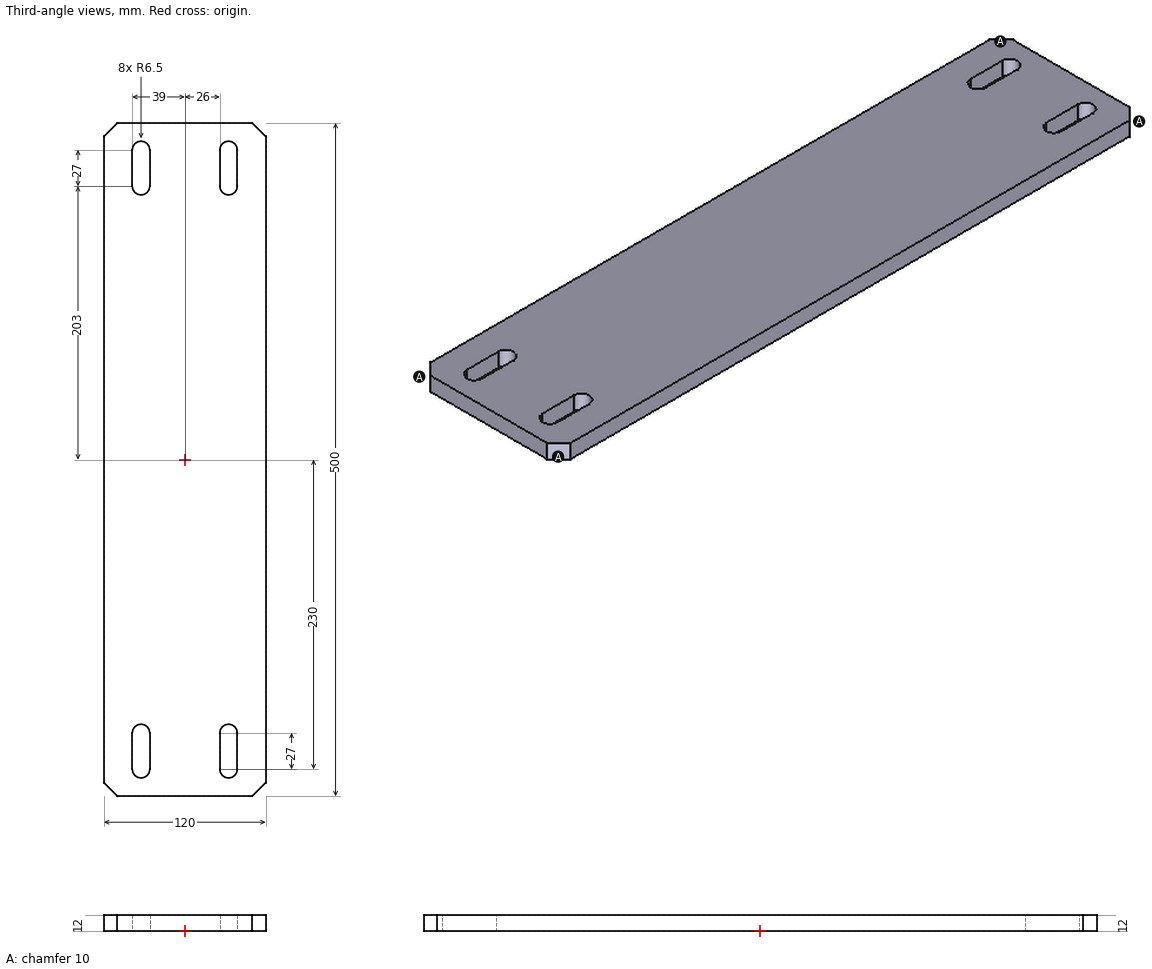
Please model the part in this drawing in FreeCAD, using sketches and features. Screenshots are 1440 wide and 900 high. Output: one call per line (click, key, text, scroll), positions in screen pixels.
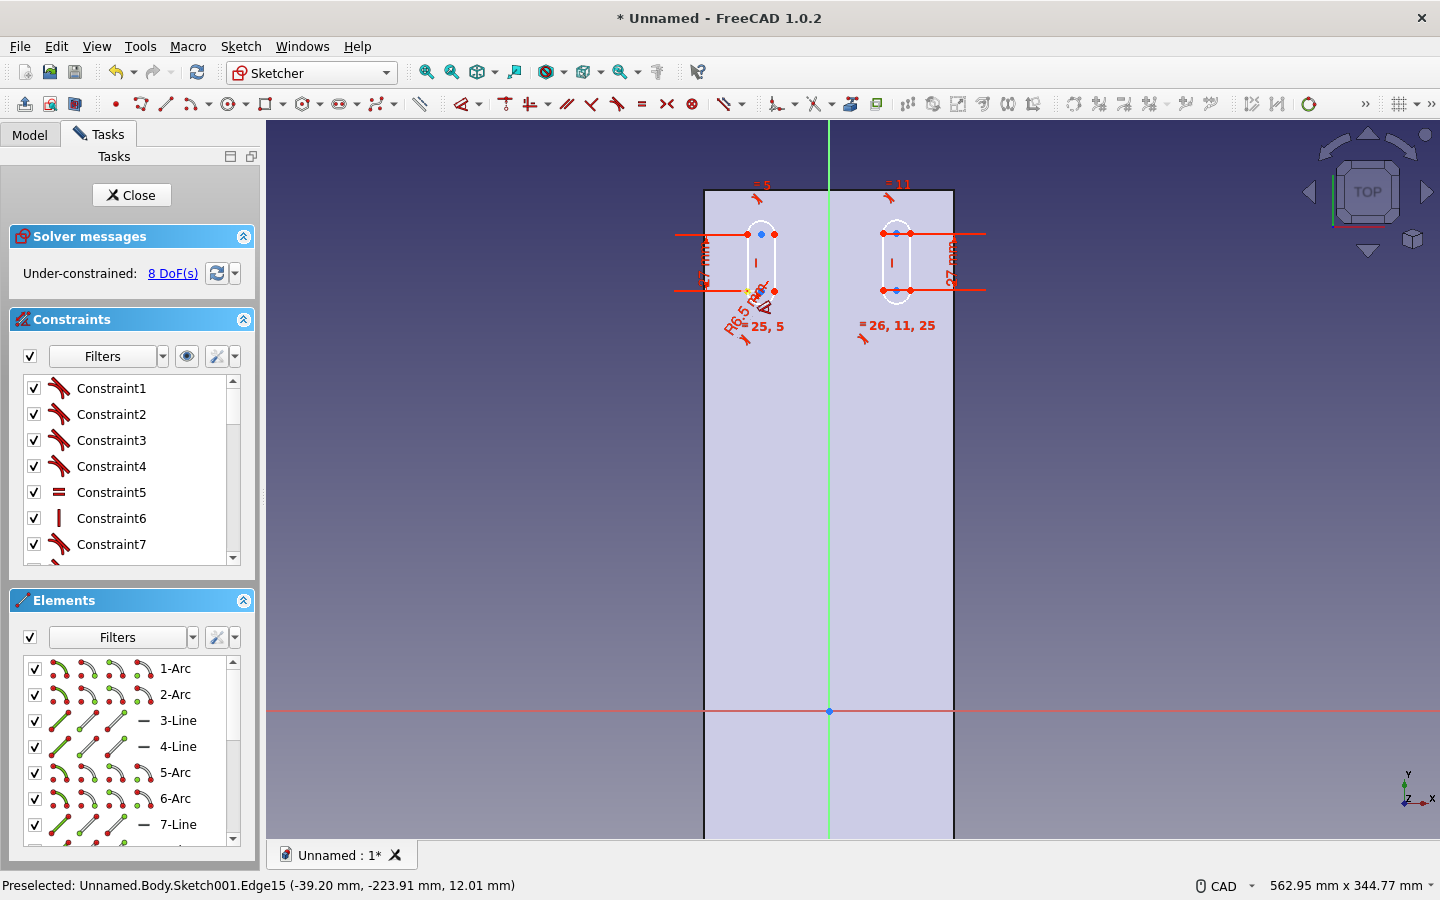
click(748, 291)
click(788, 257)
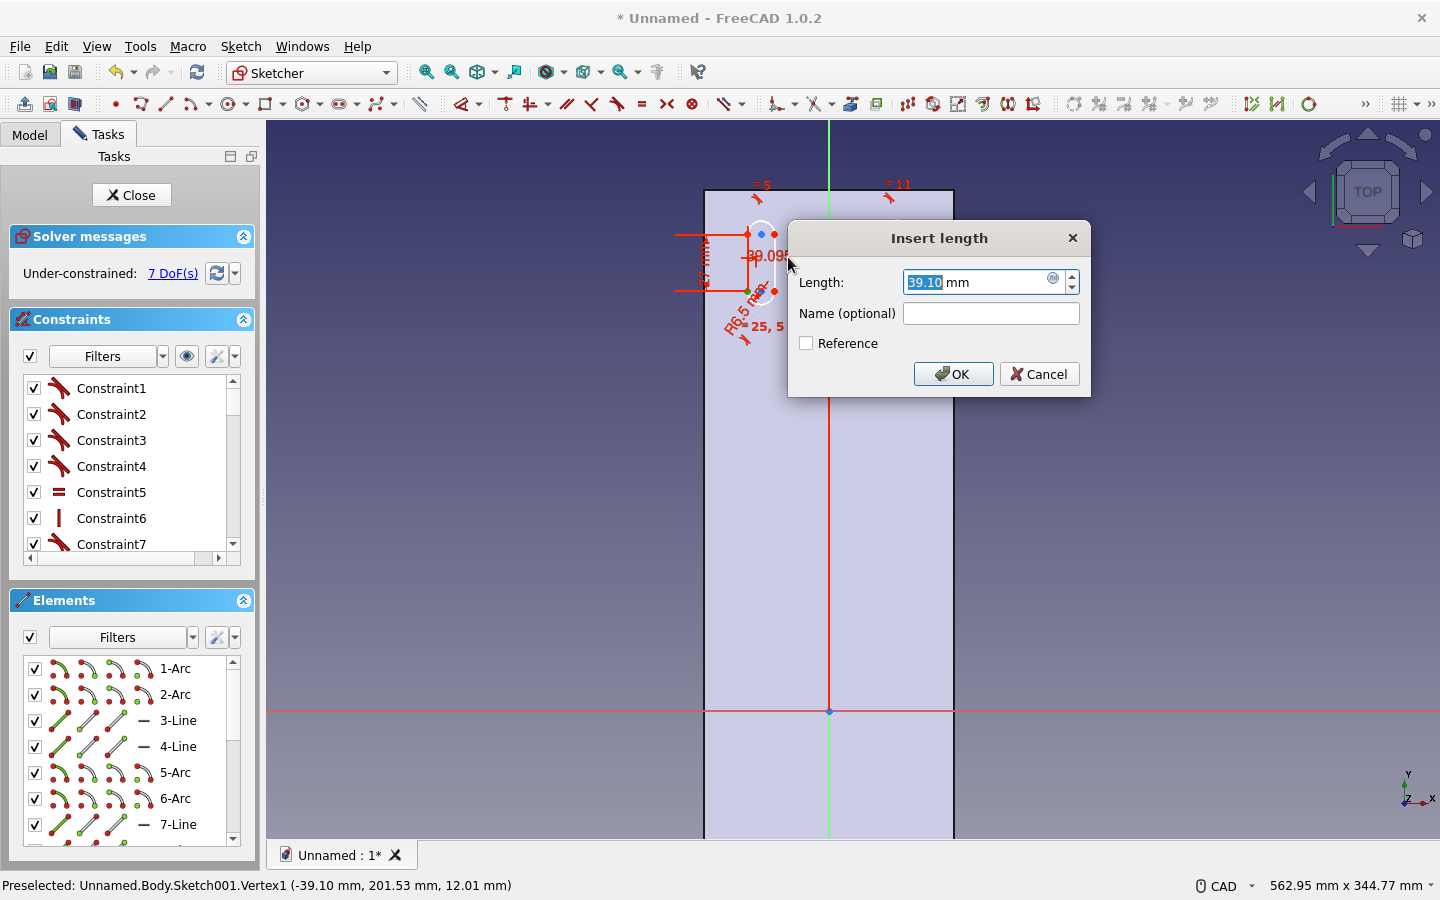
text(39)
key(Return)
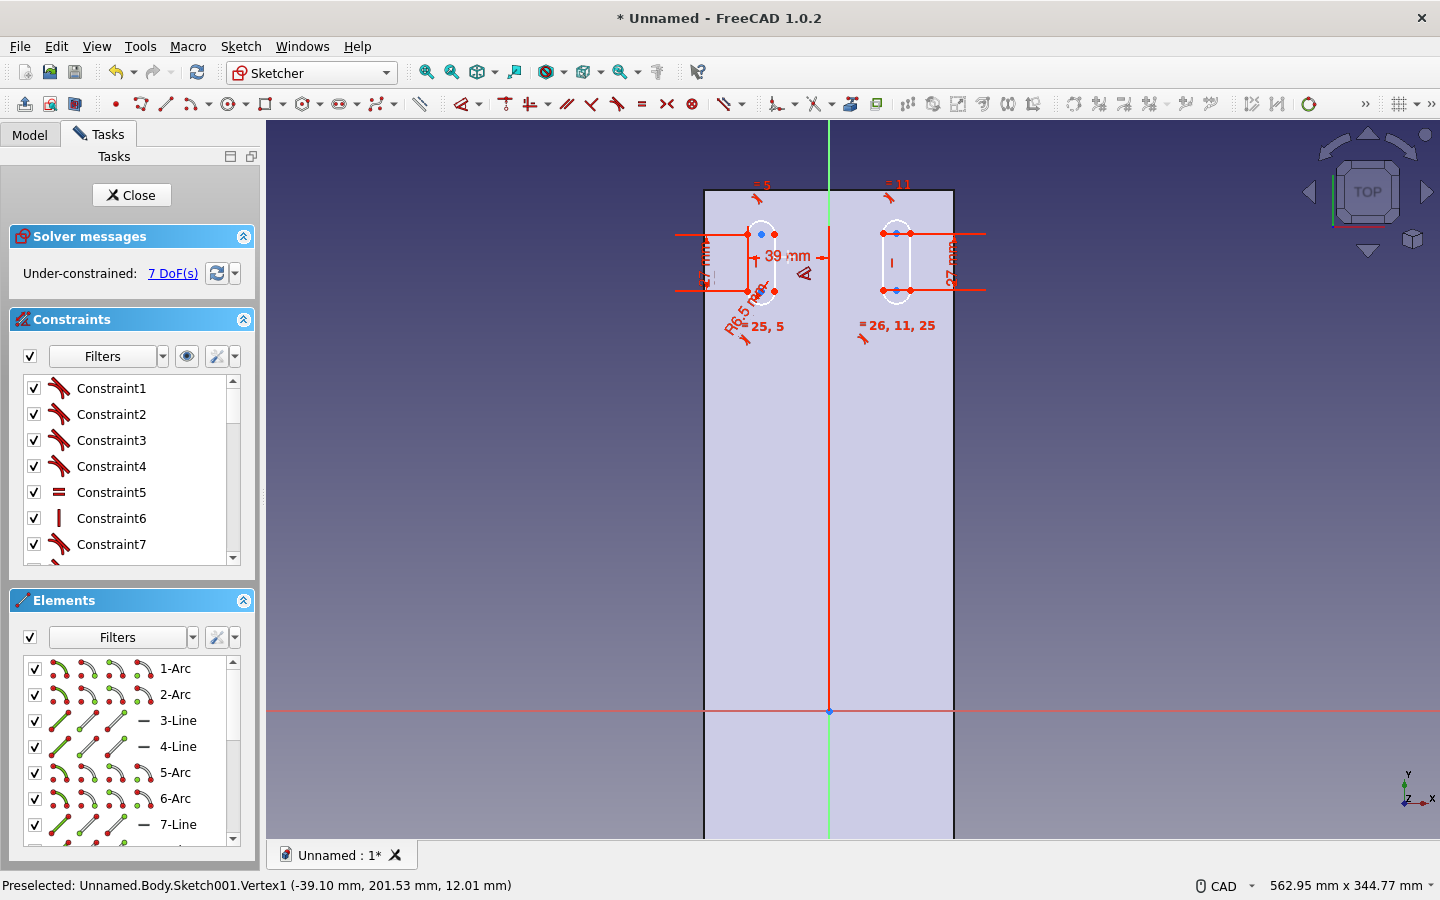
click(883, 290)
click(869, 256)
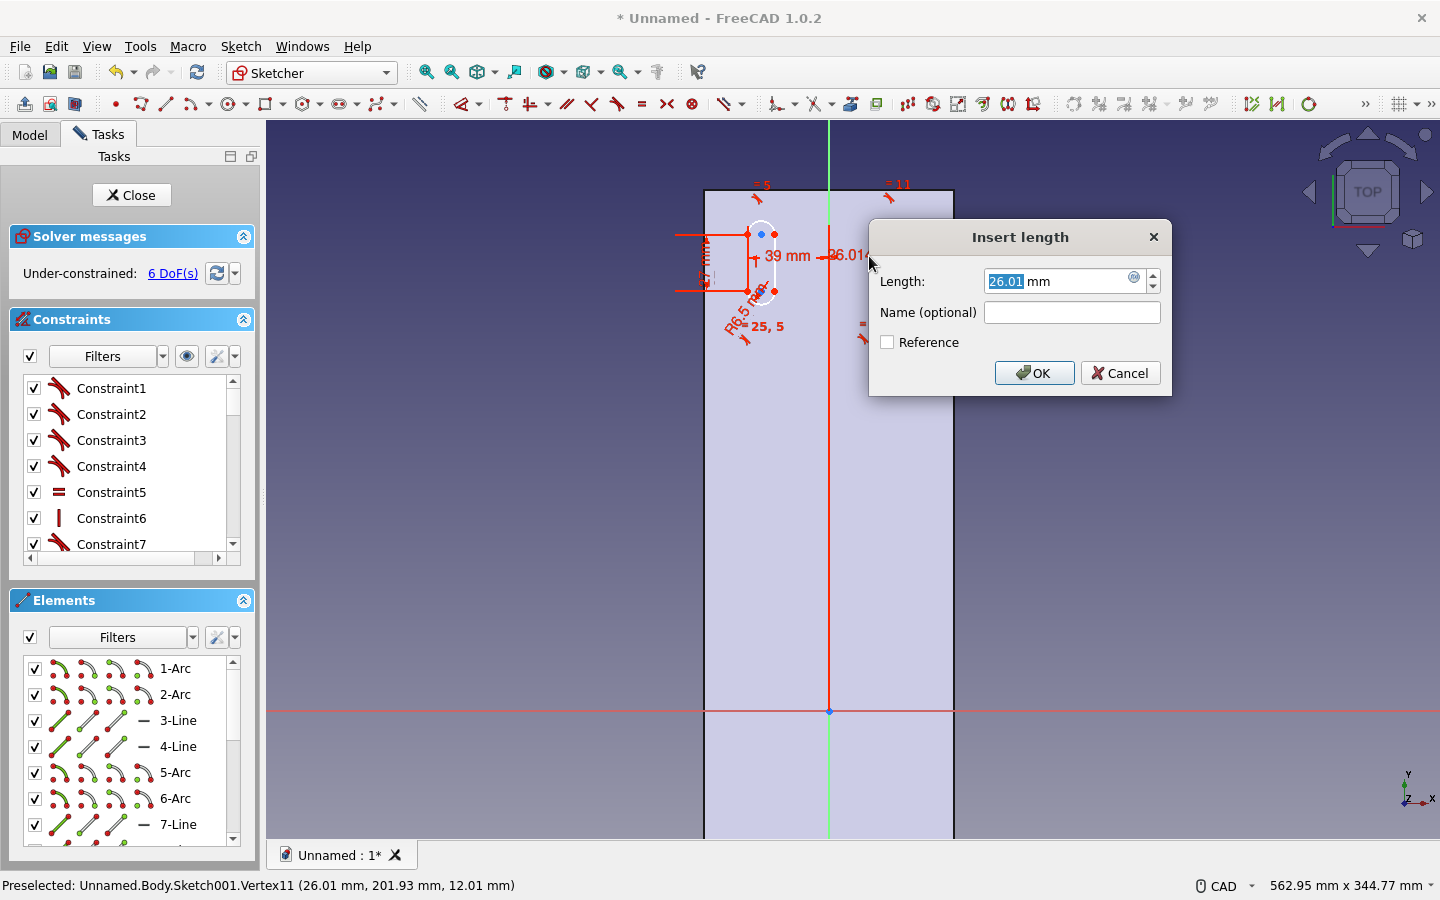
text(26)
key(Return)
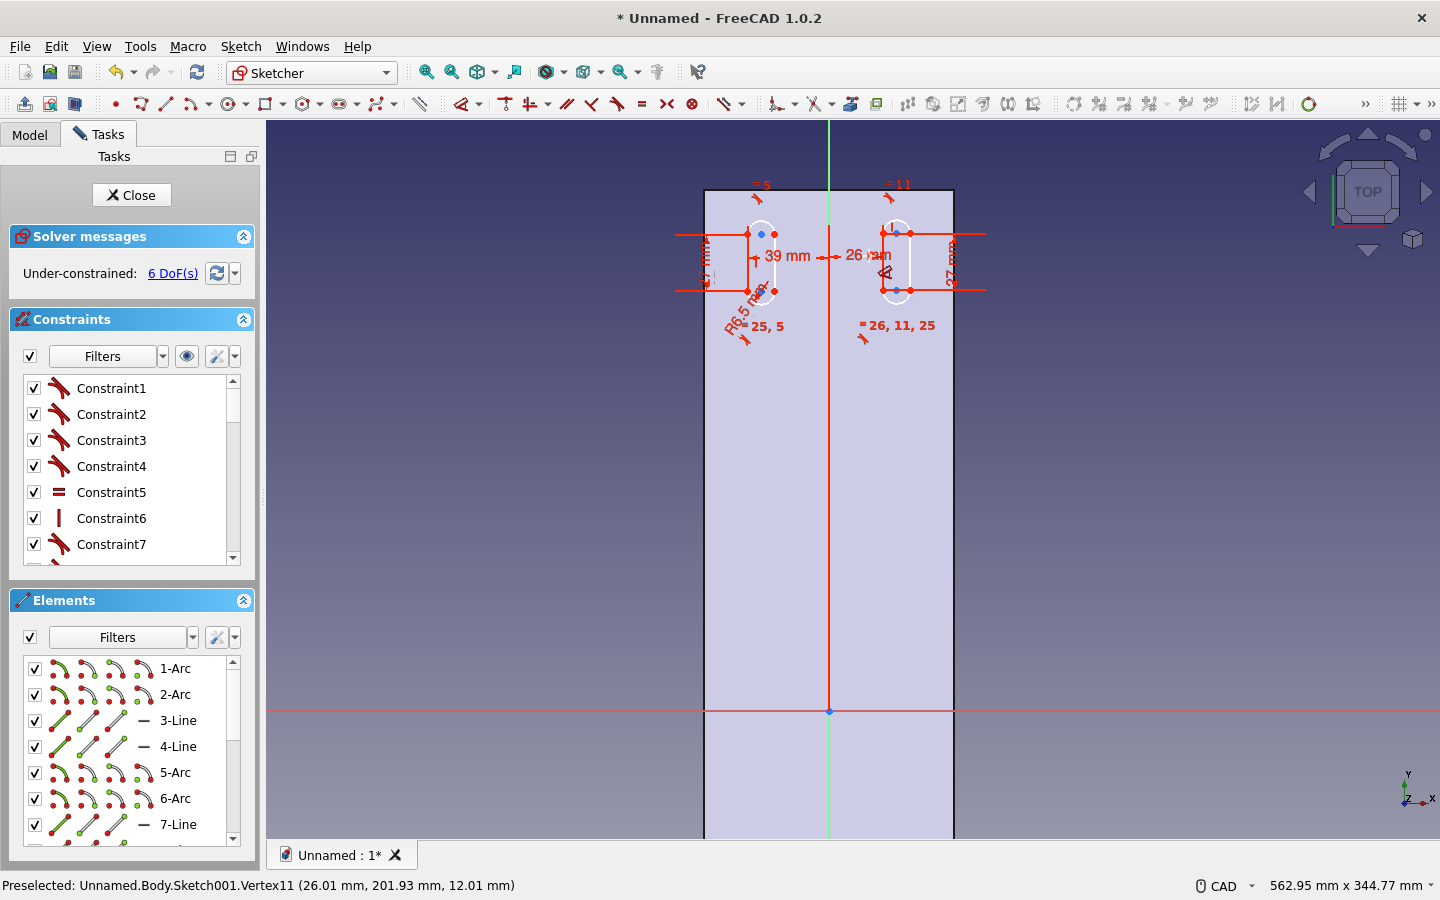
scroll(748, 290, down, 4)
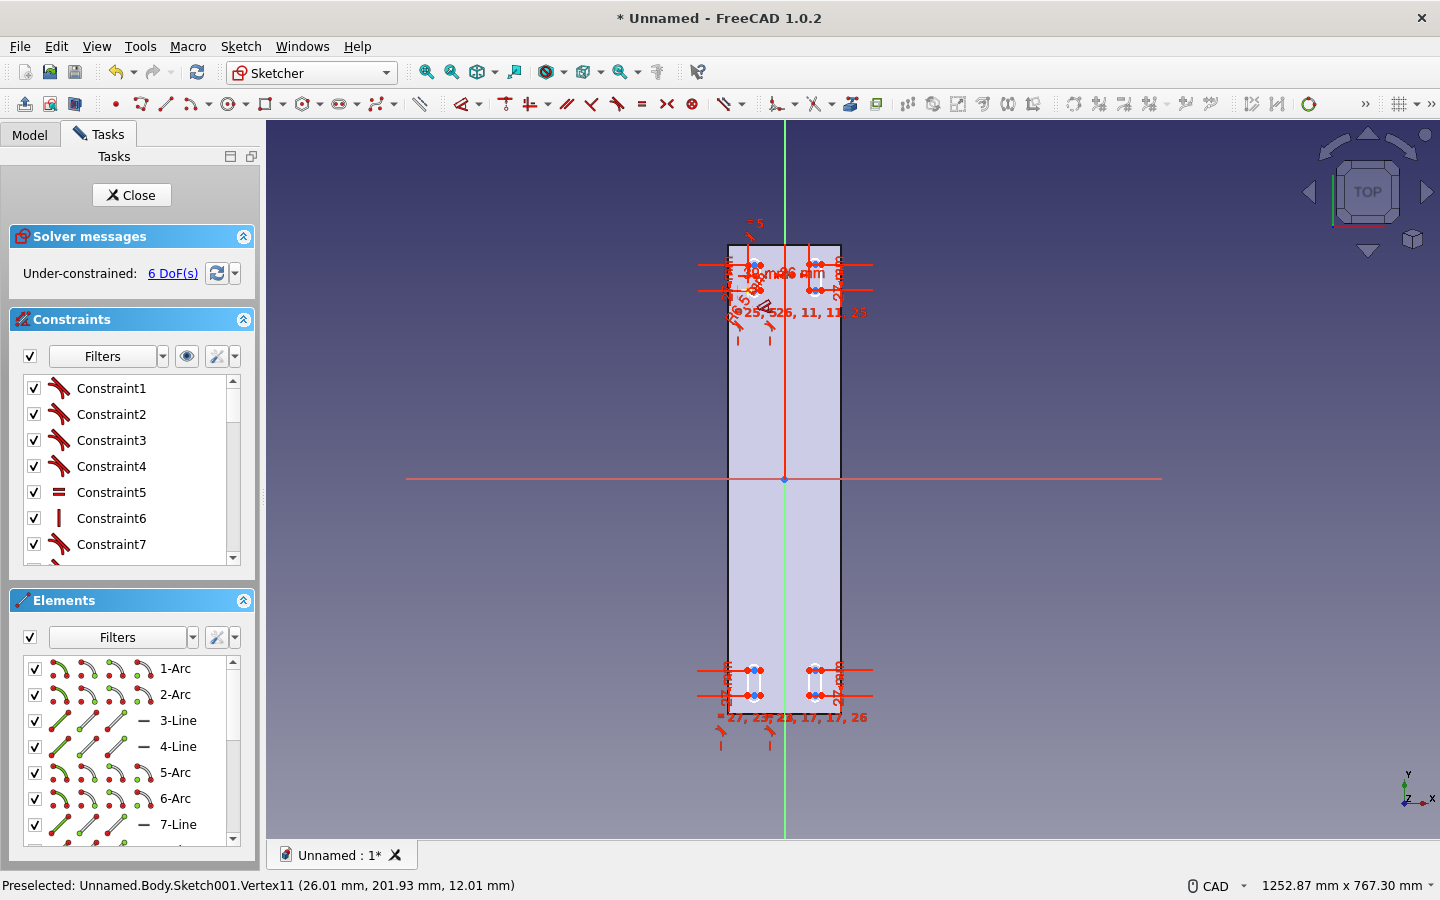
scroll(809, 696, up, 4)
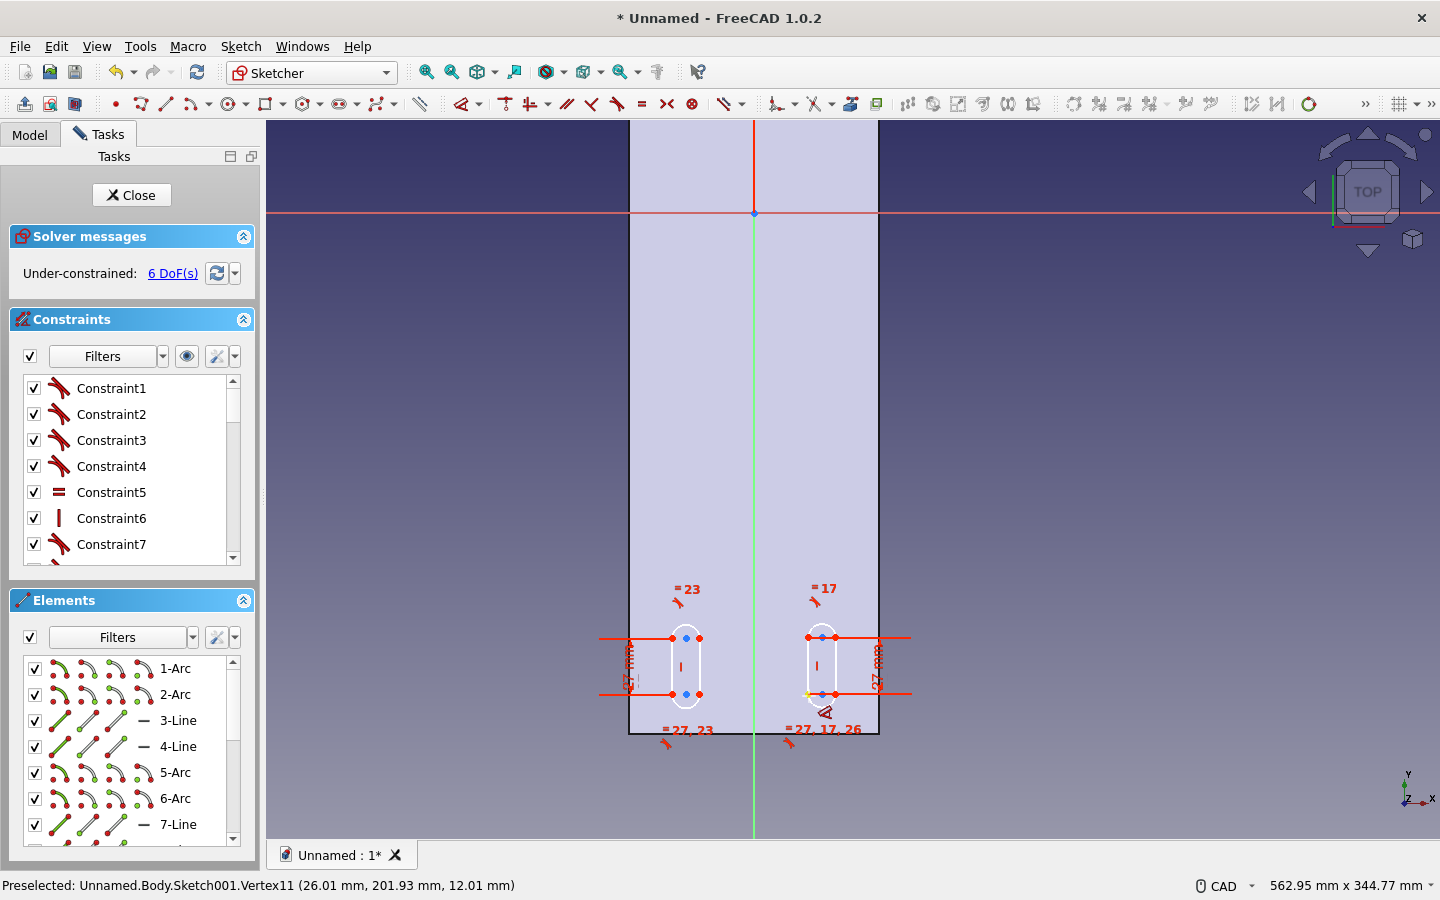
click(808, 694)
click(781, 728)